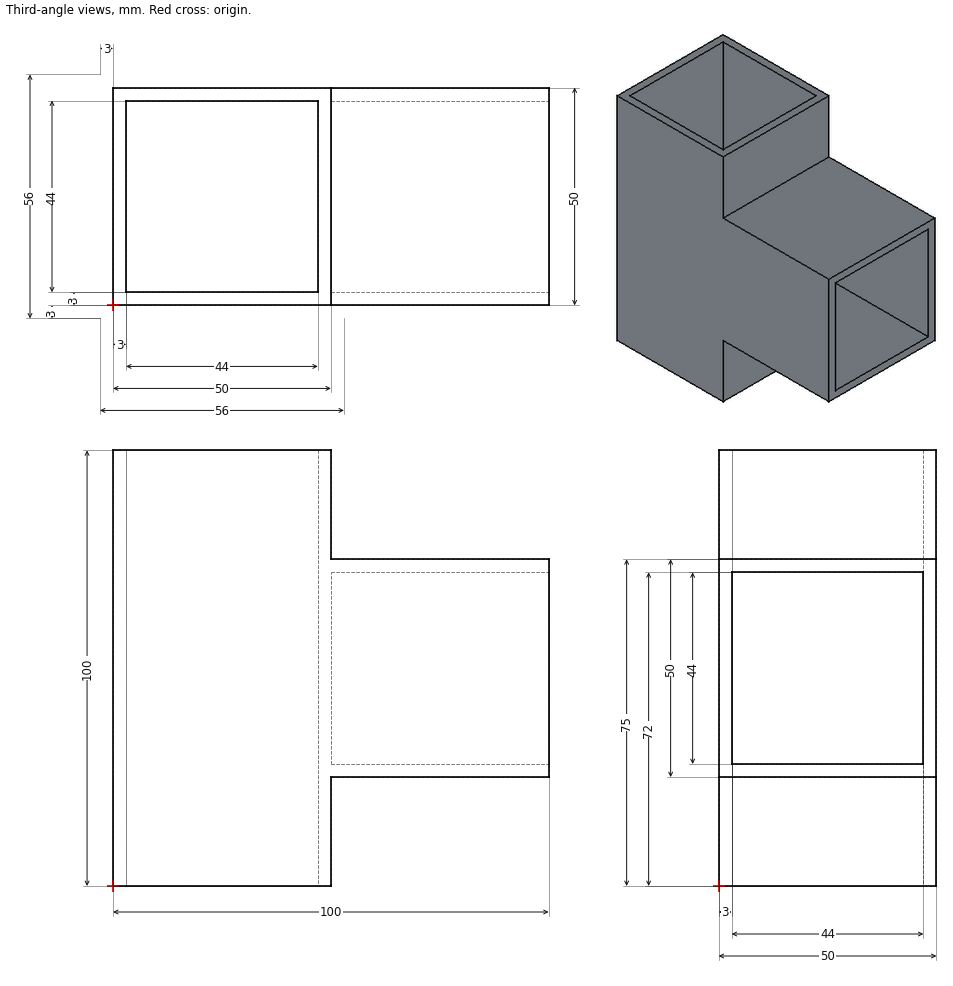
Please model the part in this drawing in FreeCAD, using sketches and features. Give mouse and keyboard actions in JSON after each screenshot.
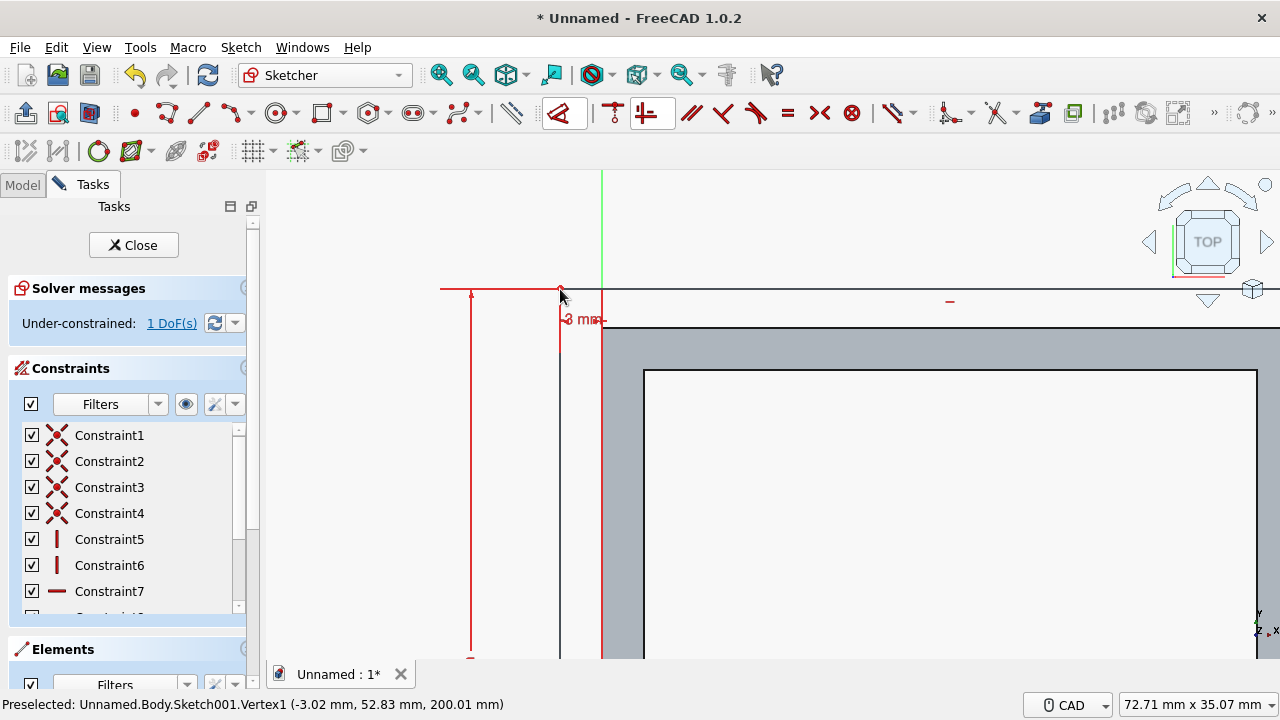
{"action": "scroll", "coordinate": [561, 262], "scroll_direction": "down", "scroll_amount": 5}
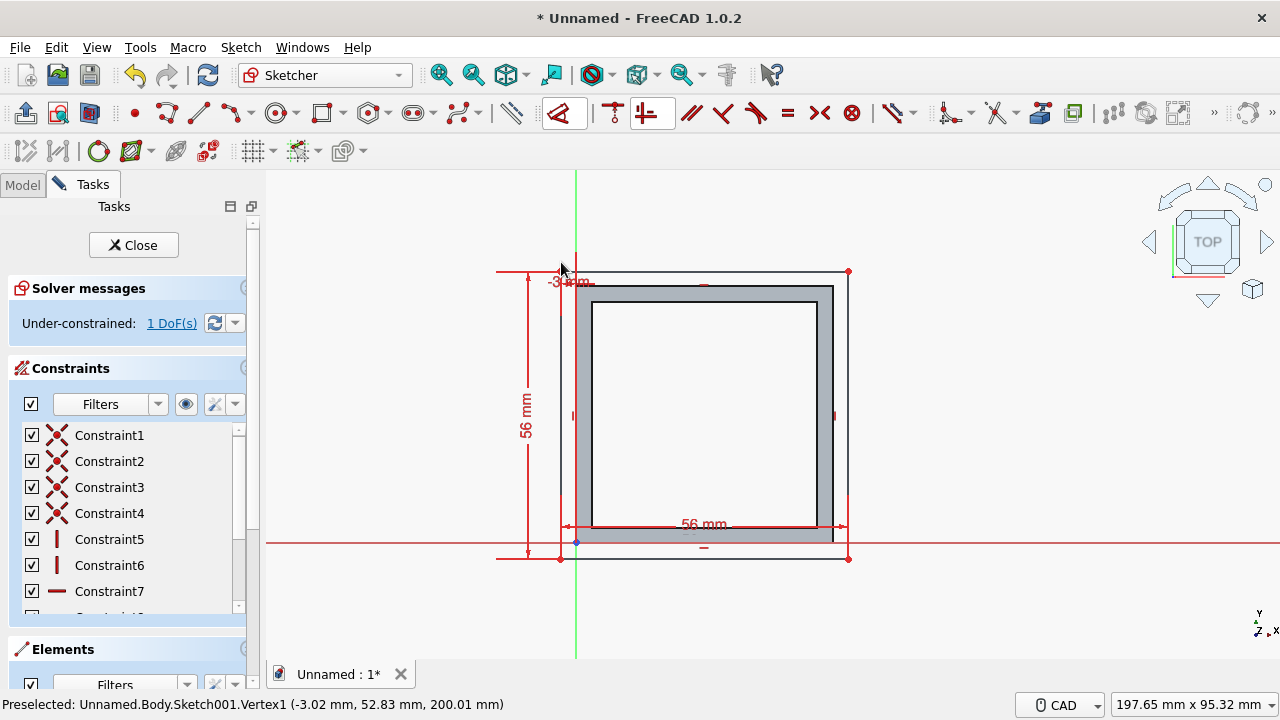
{"action": "scroll", "coordinate": [561, 559], "scroll_direction": "up", "scroll_amount": 5}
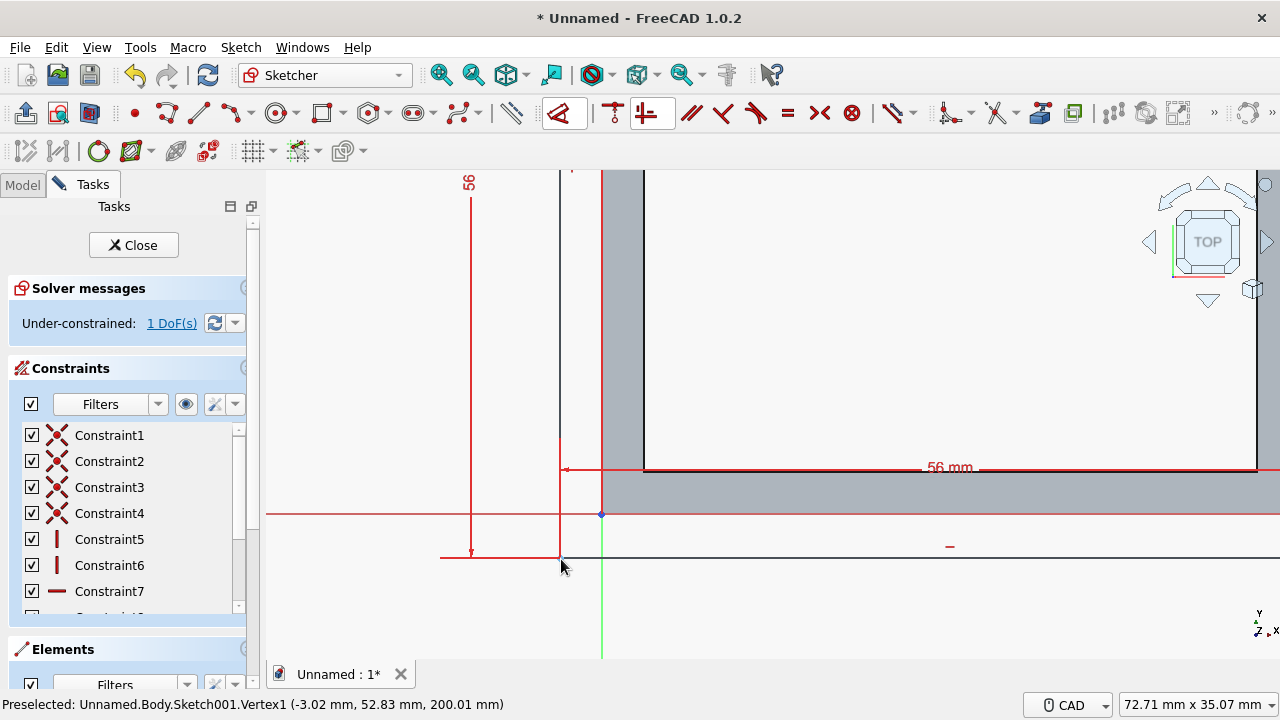
{"action": "left_click", "coordinate": [560, 558]}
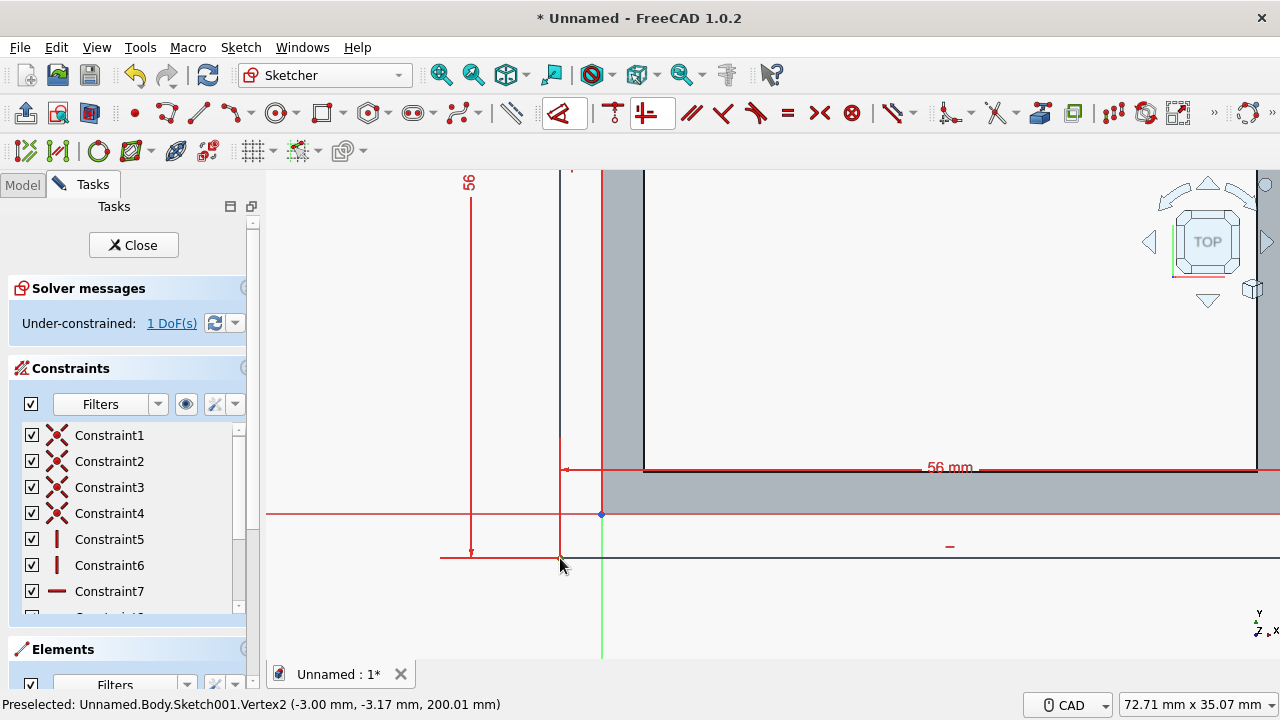
{"action": "left_click", "coordinate": [582, 114]}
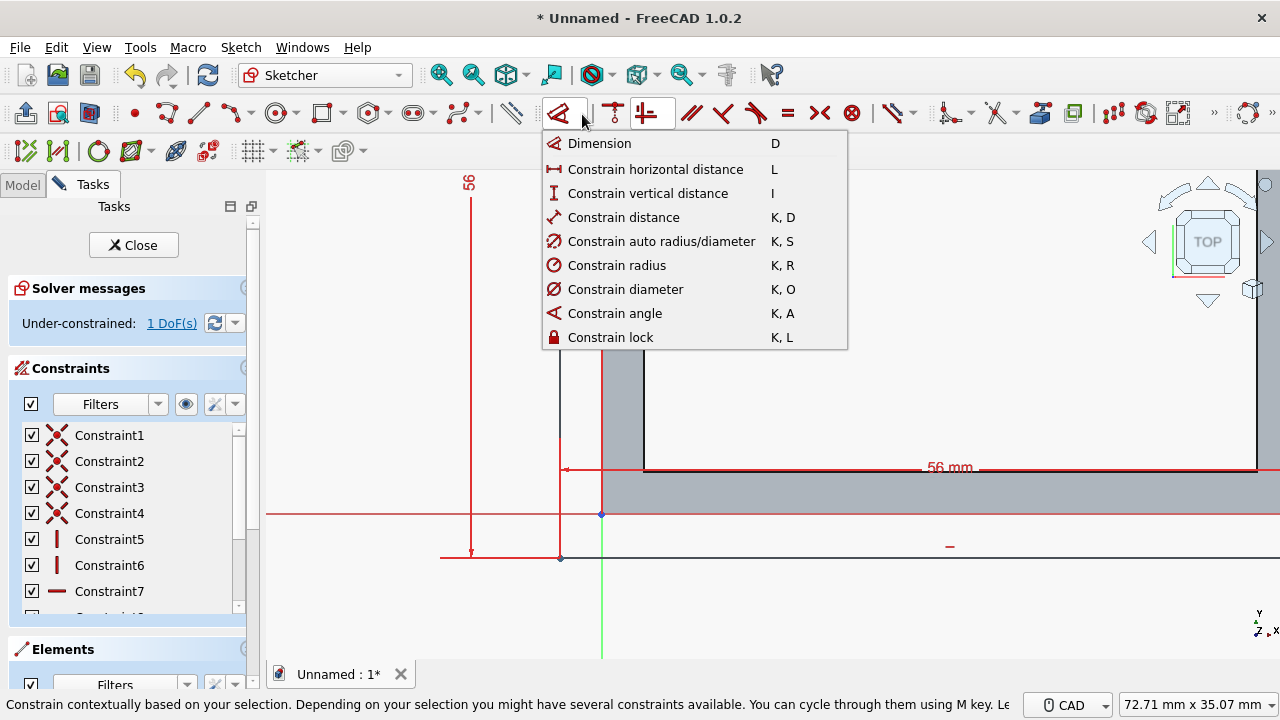
{"action": "left_click", "coordinate": [695, 193]}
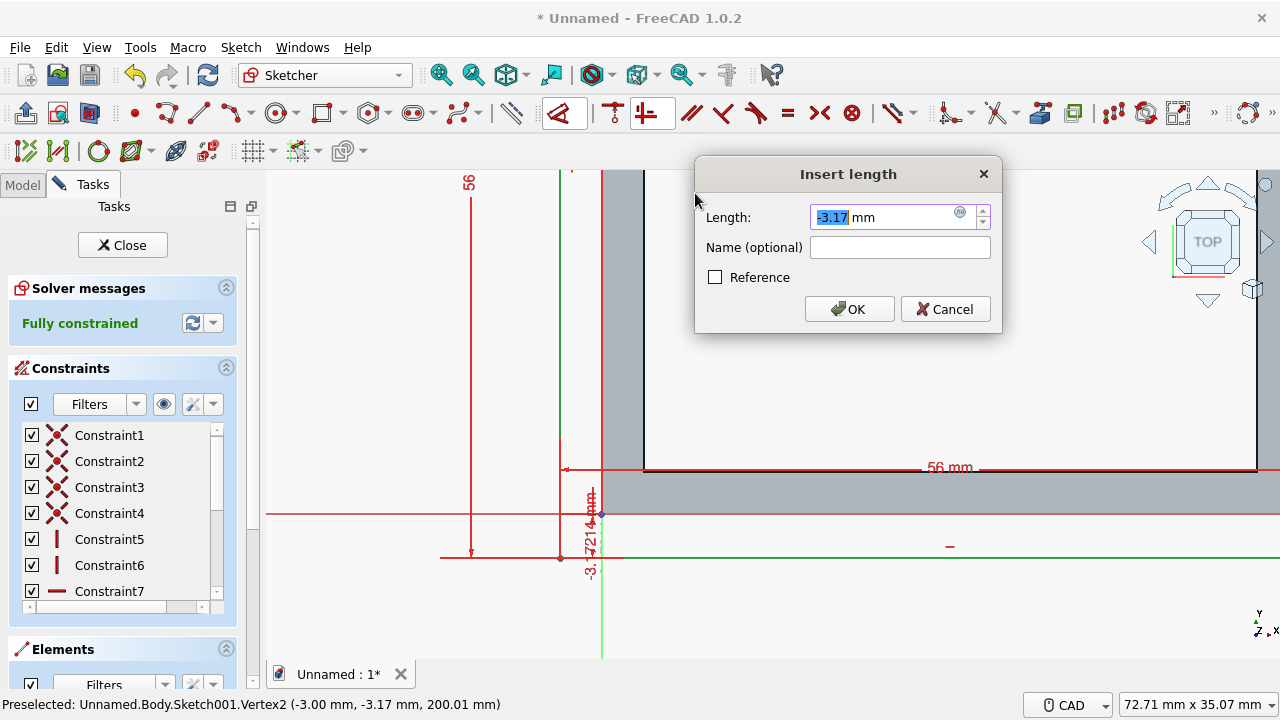
{"action": "type", "text": "-3"}
{"action": "key", "text": "Return"}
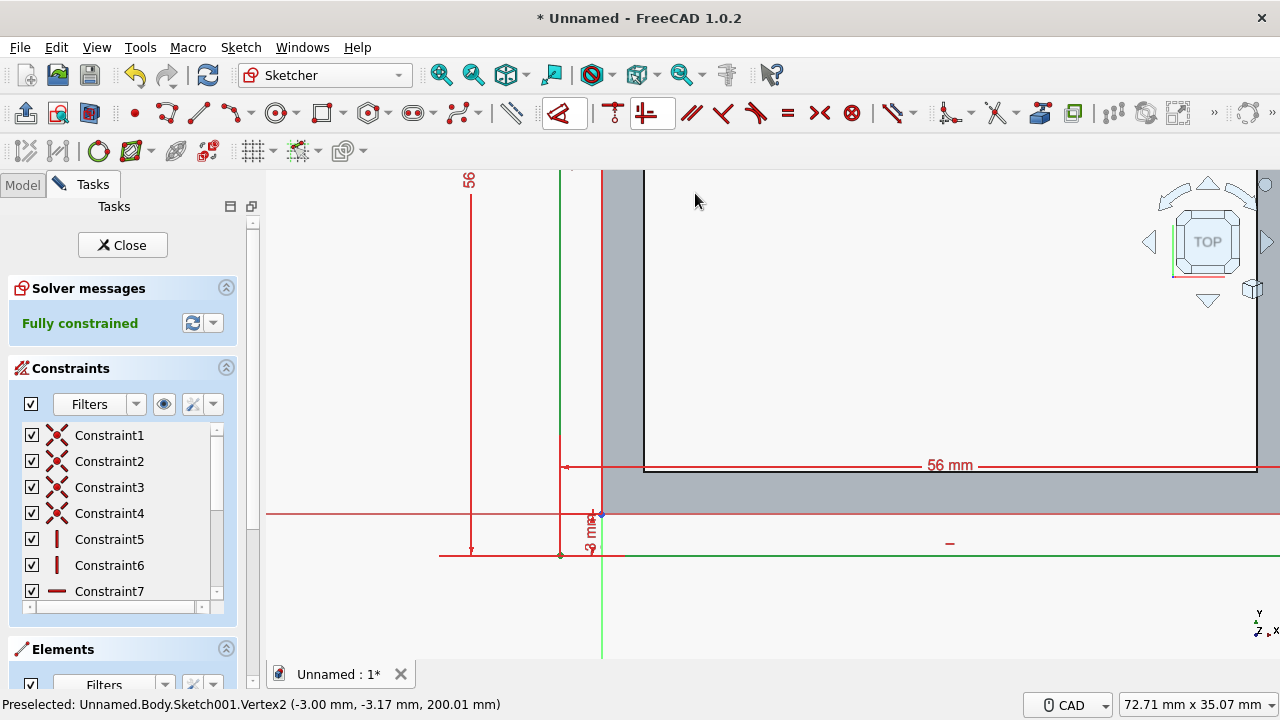
{"action": "left_click", "coordinate": [123, 245]}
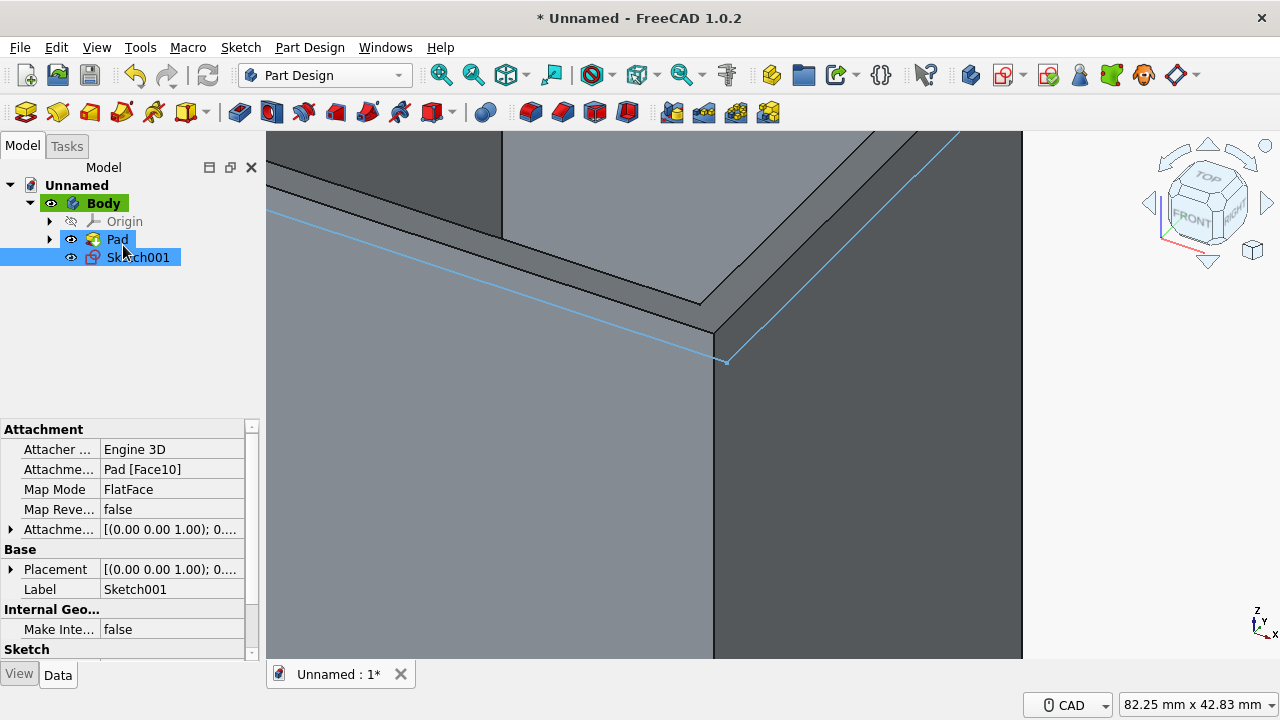
{"action": "left_click", "coordinate": [240, 112]}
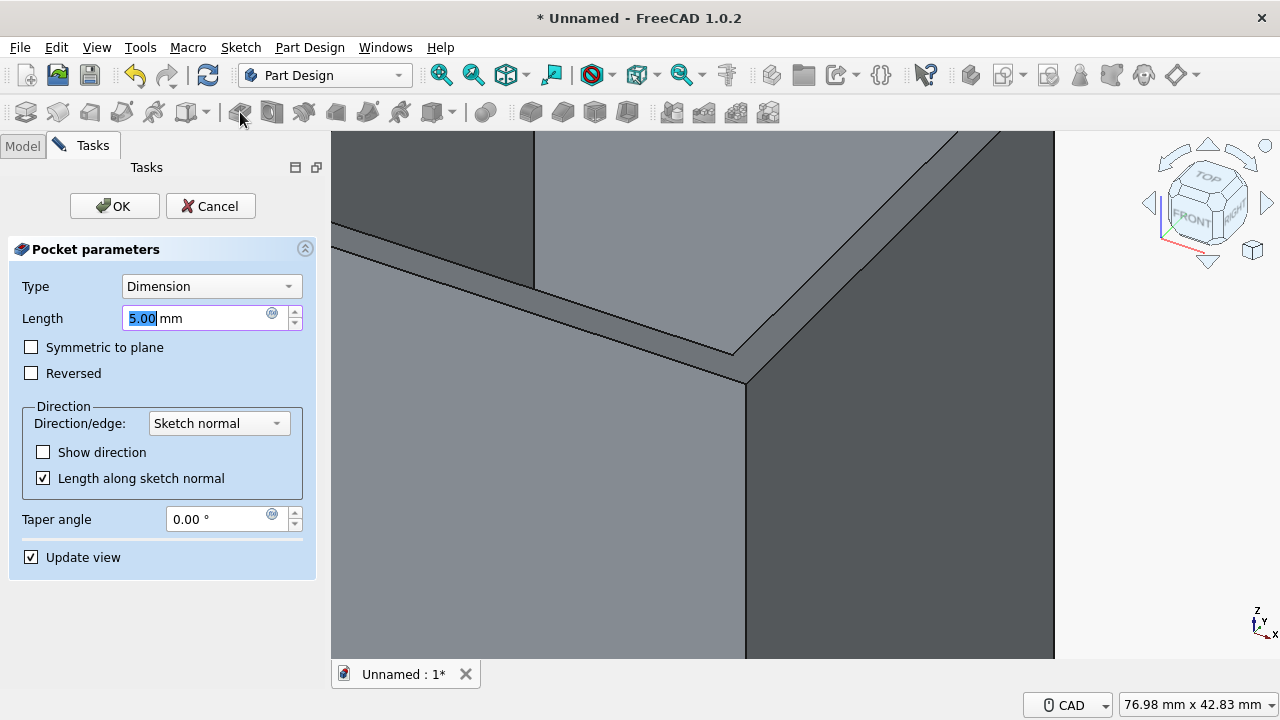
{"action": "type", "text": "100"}
{"action": "key", "text": "Tab"}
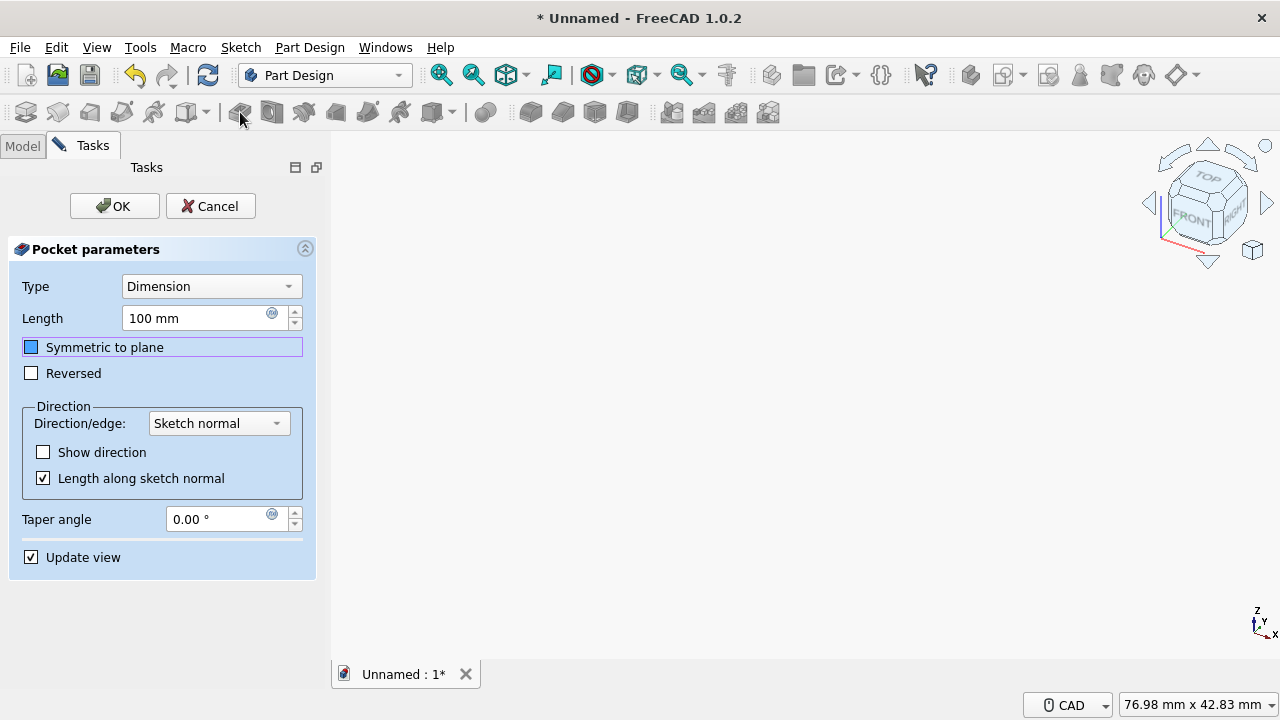
{"action": "left_click", "coordinate": [115, 206]}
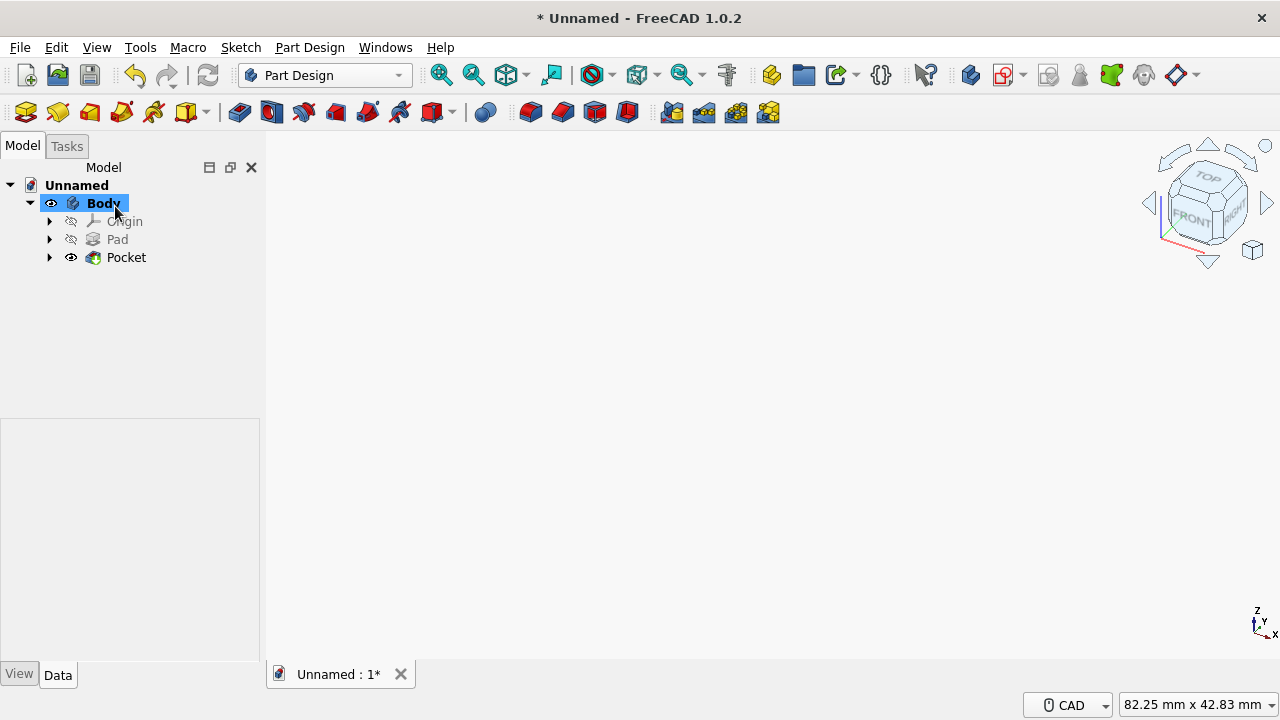
{"action": "key", "text": "v f"}